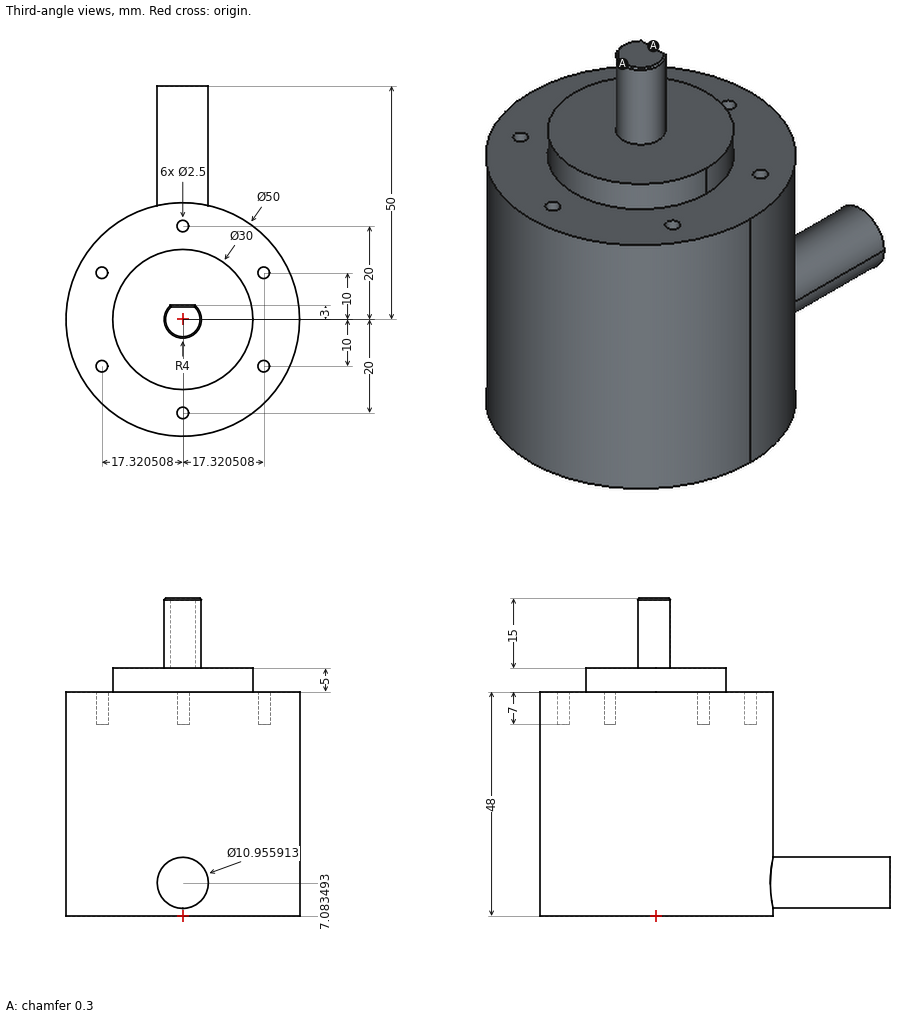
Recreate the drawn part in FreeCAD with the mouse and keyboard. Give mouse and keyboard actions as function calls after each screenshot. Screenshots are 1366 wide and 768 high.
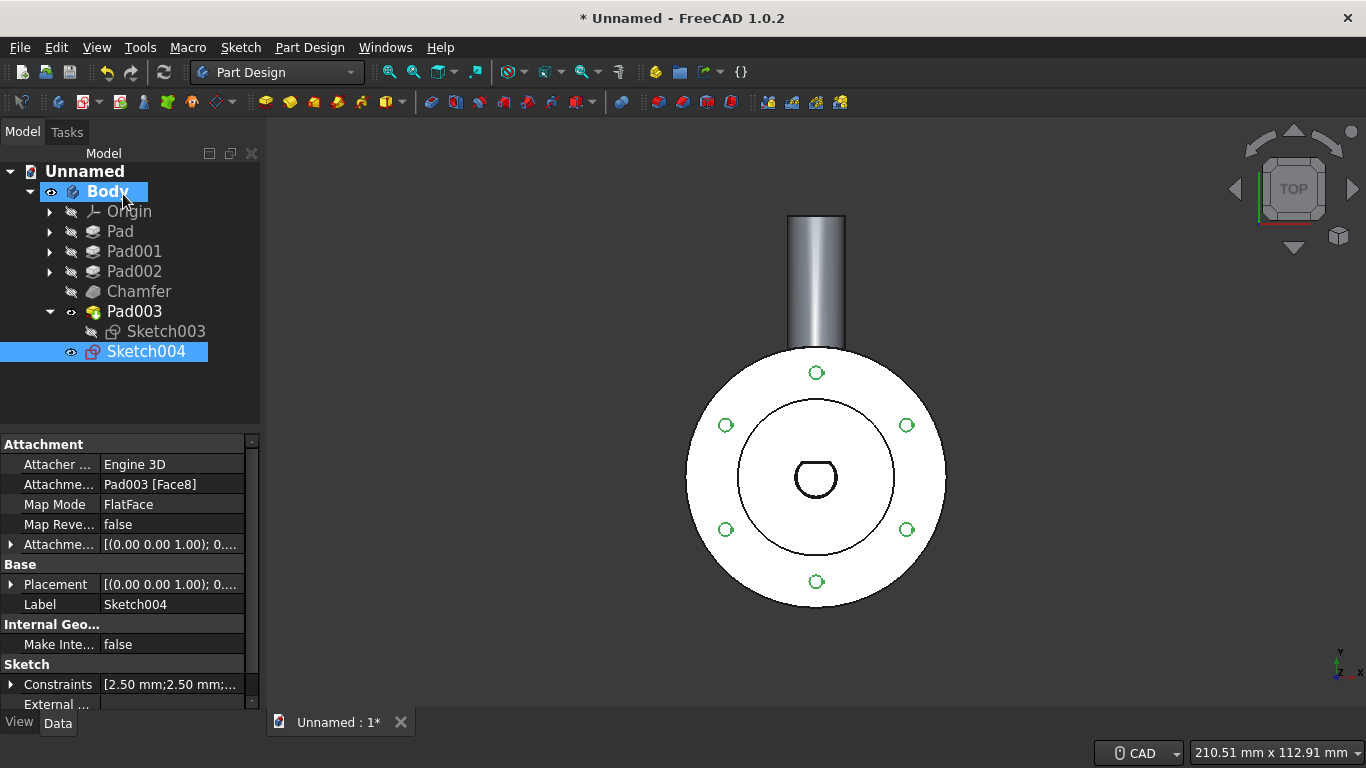
click(432, 102)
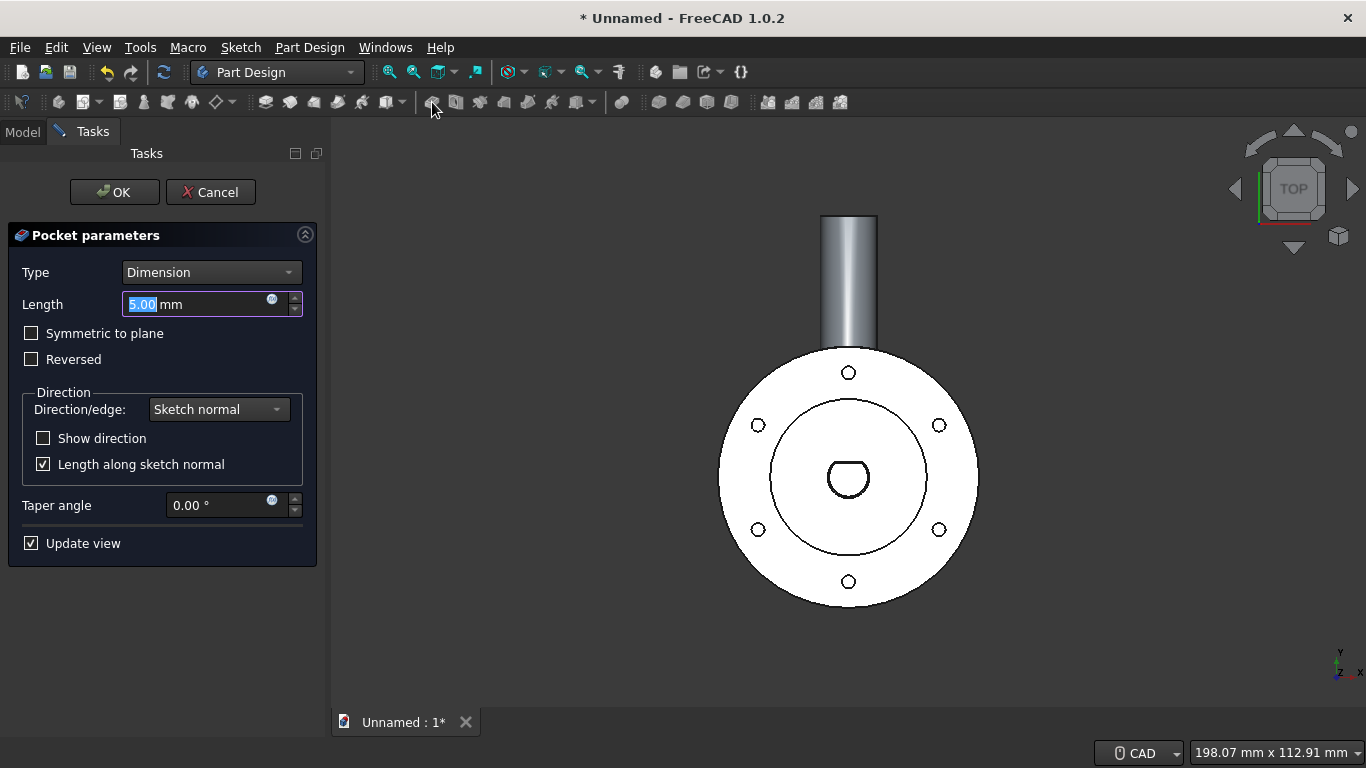
text(7)
key(Tab)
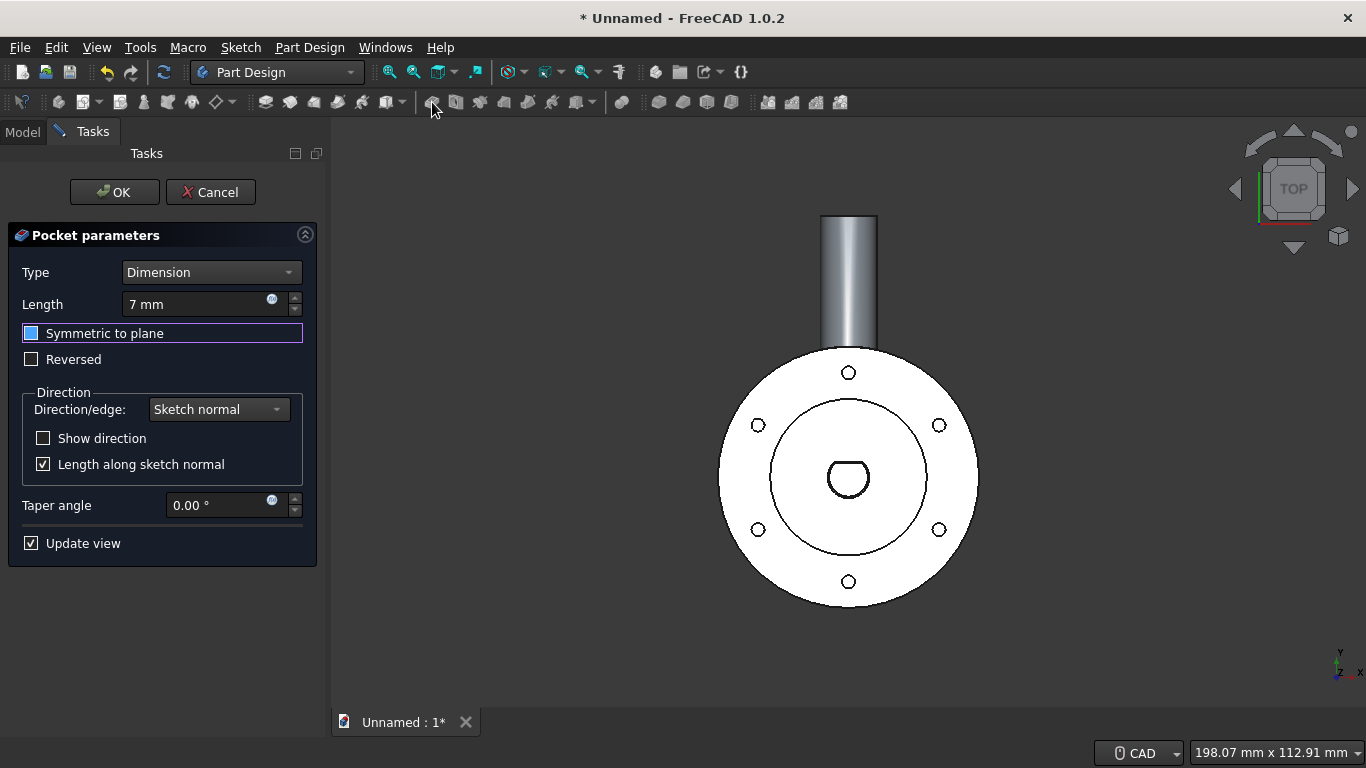
click(115, 192)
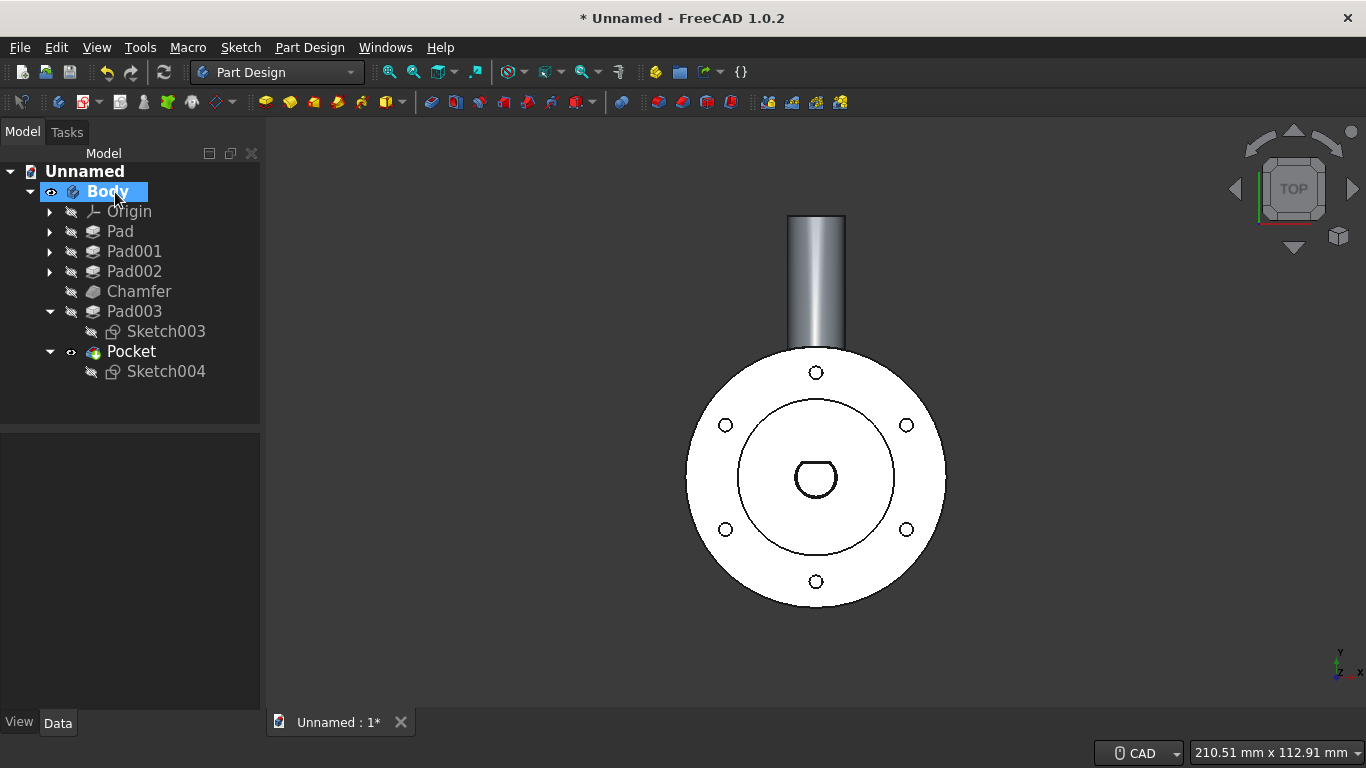
key(0)